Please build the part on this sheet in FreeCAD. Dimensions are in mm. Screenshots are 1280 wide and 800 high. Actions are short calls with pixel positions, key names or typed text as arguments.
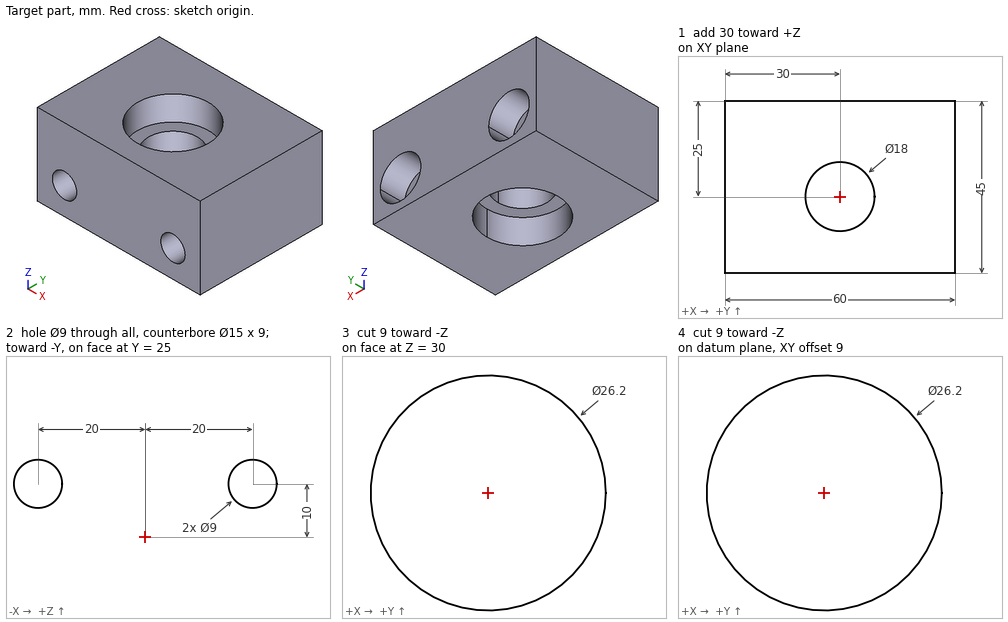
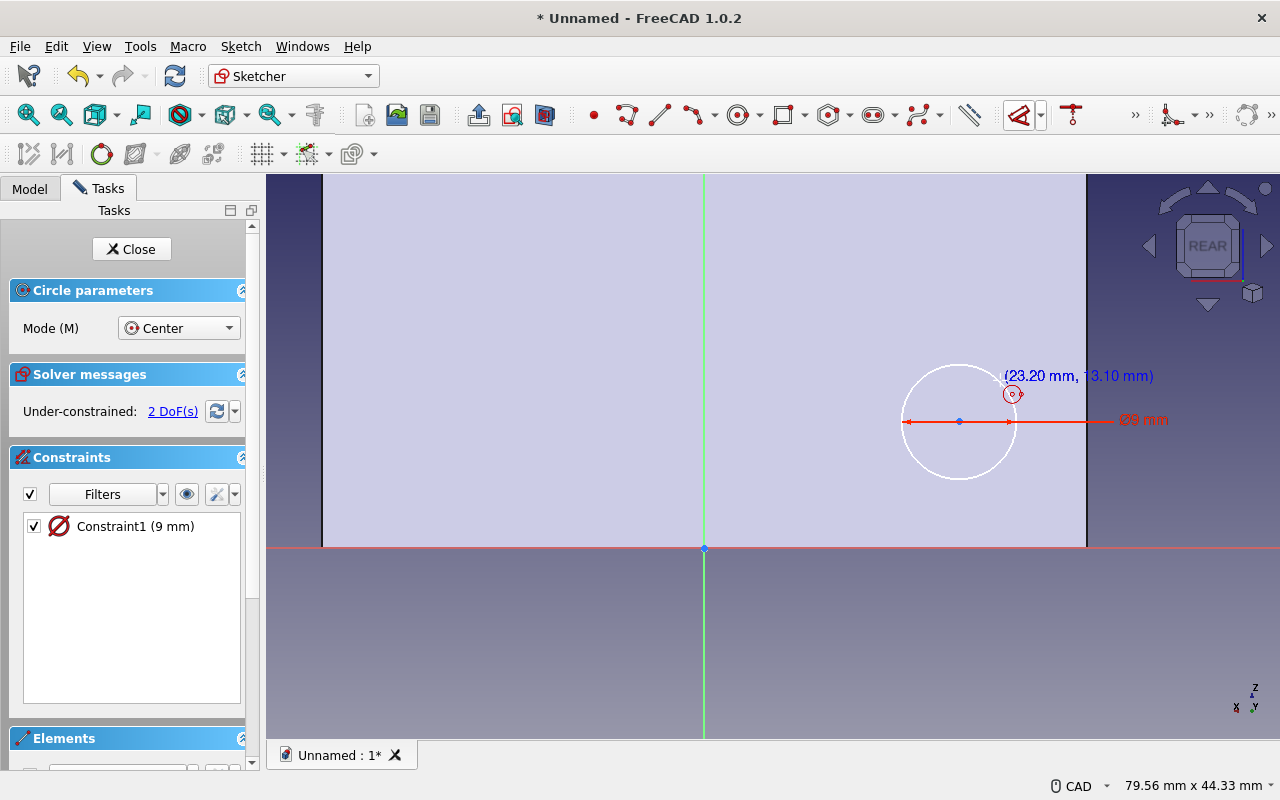
click(449, 421)
move(490, 380)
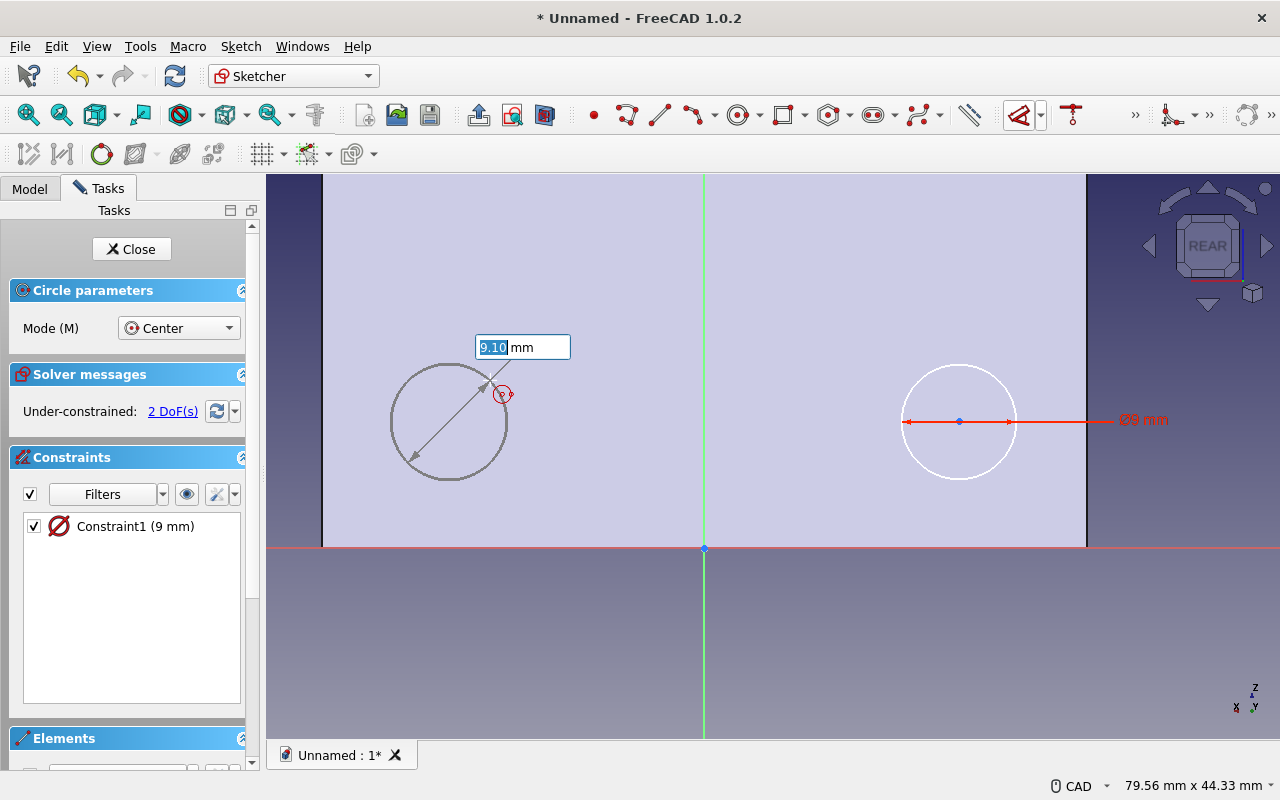
text(9)
key(Return)
key(Escape)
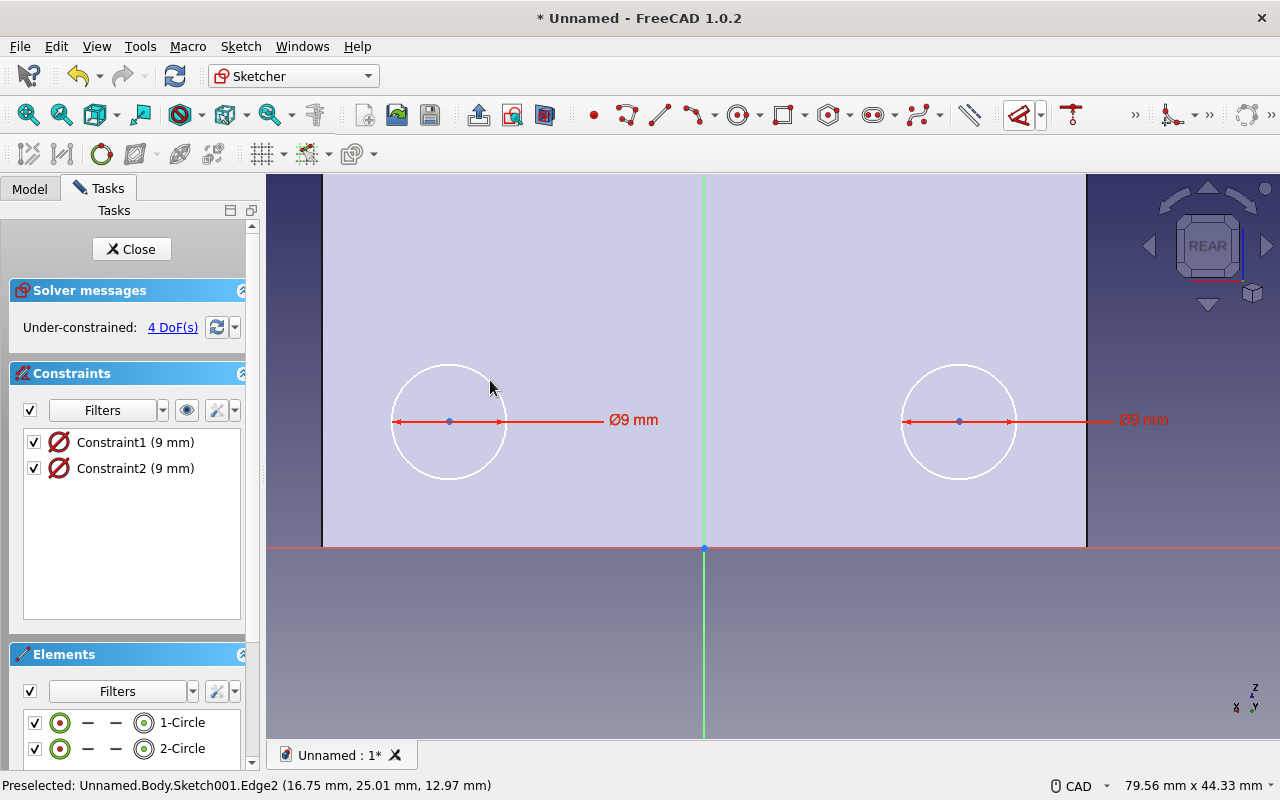
click(959, 422)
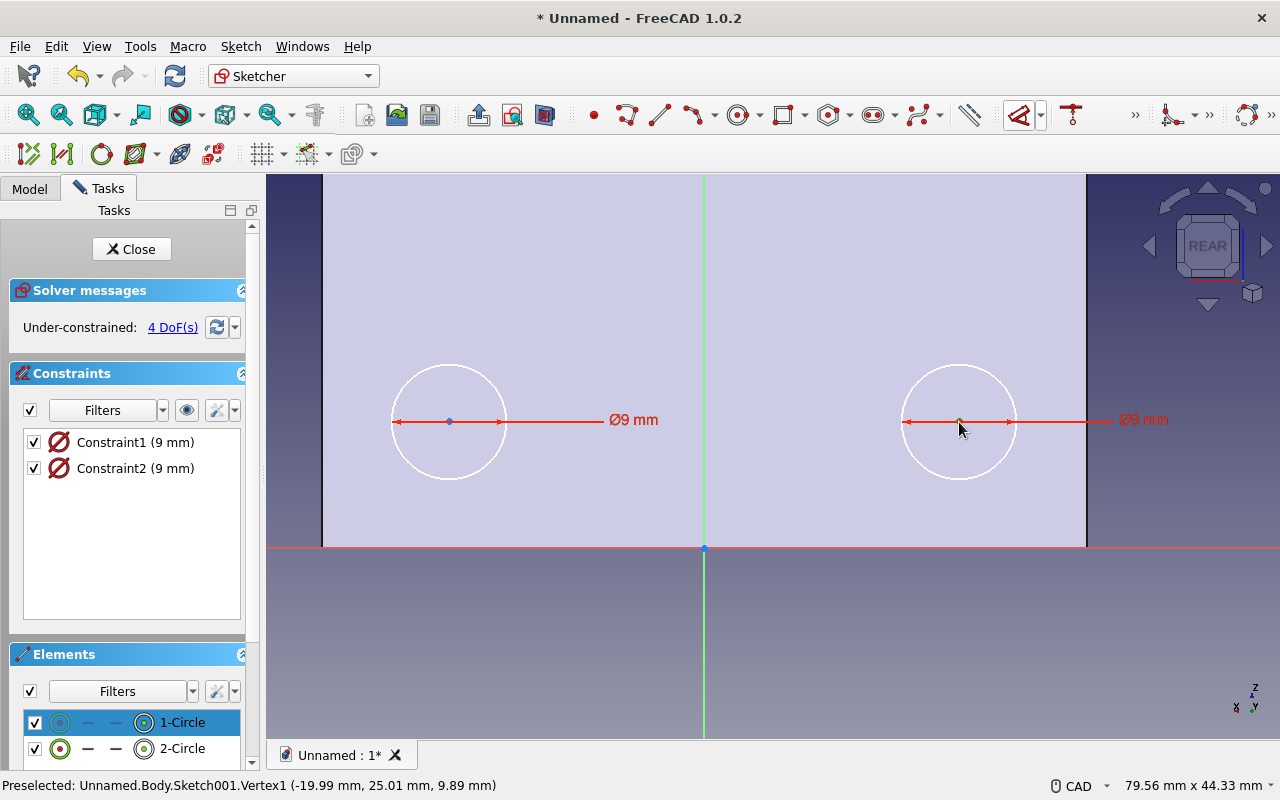
click(449, 422)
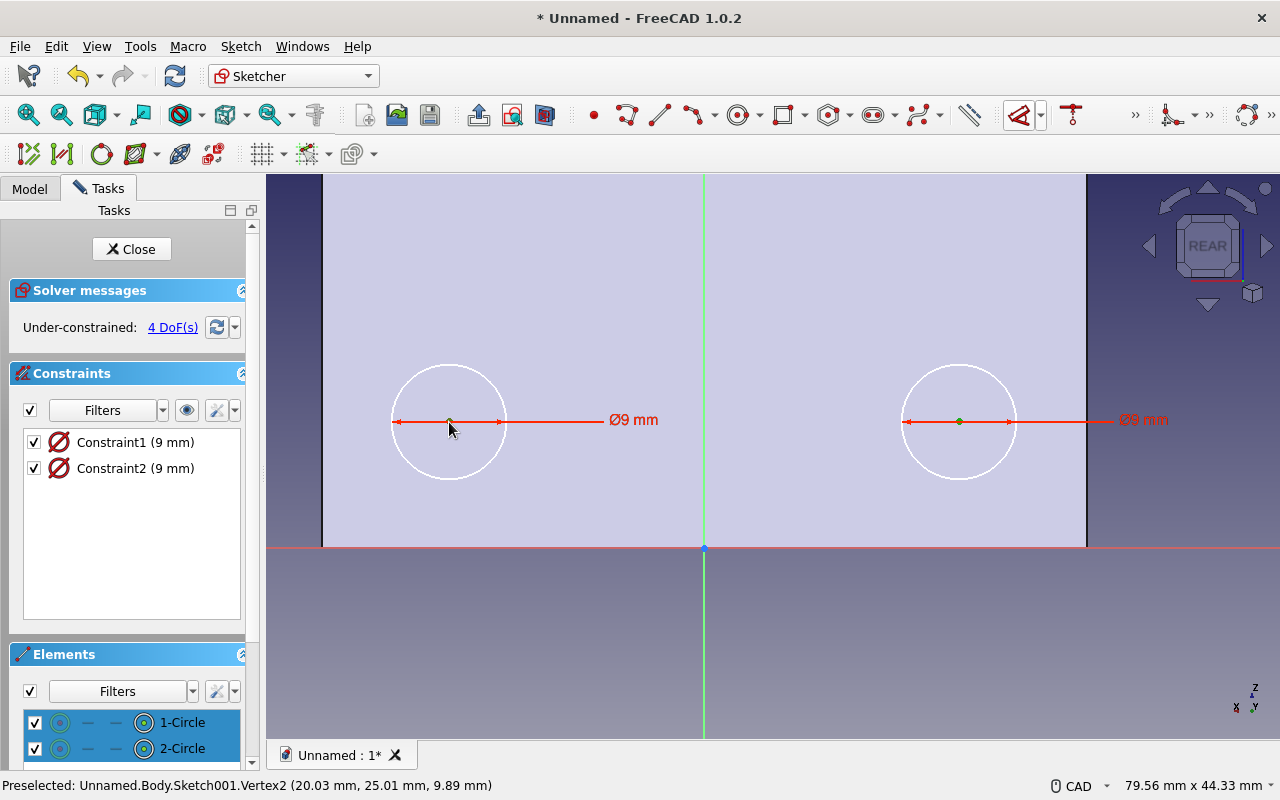
key(h)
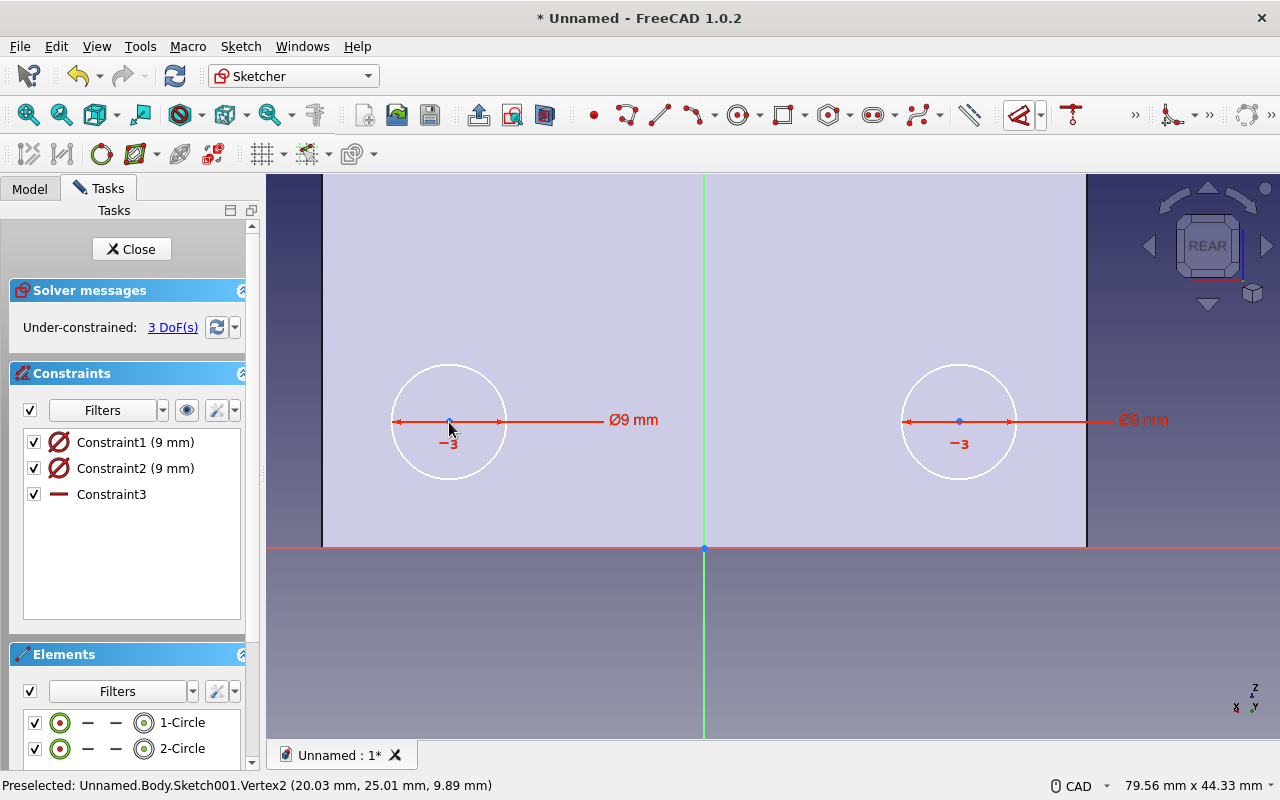
click(959, 422)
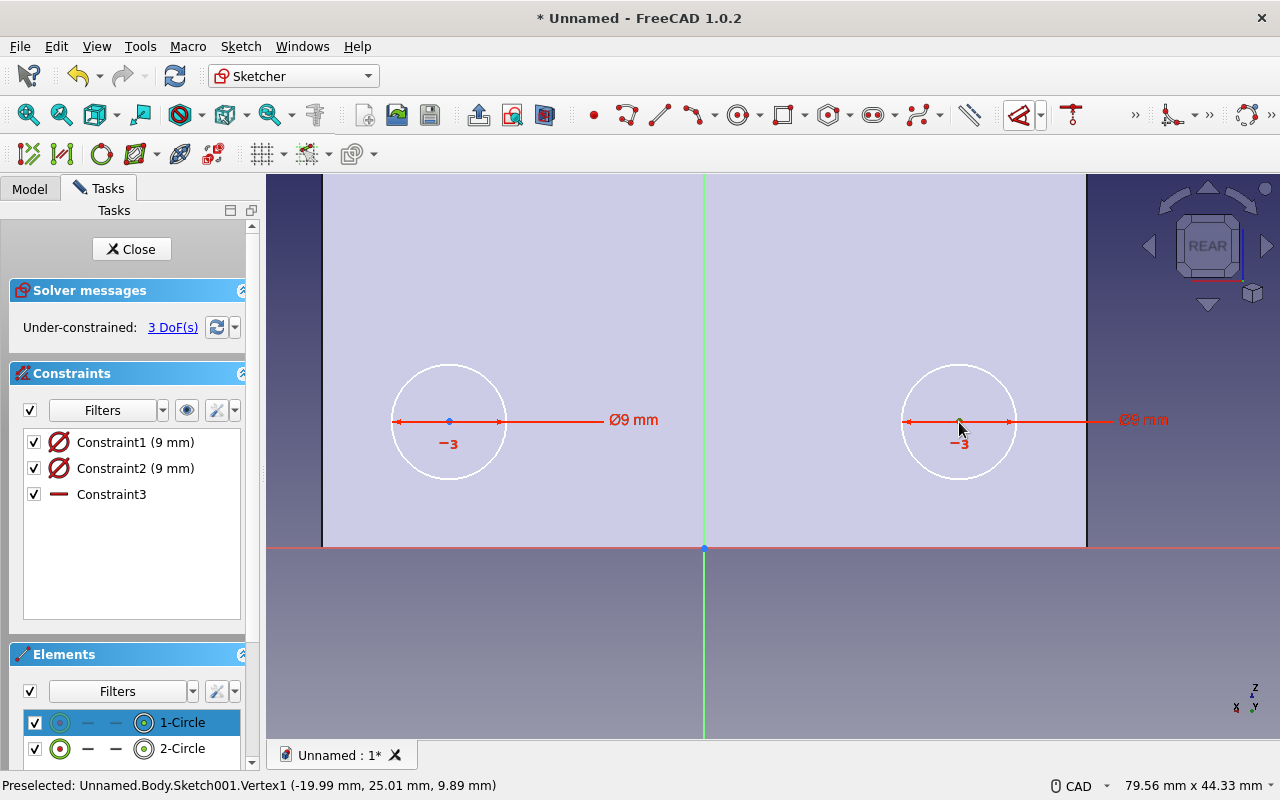
key(l)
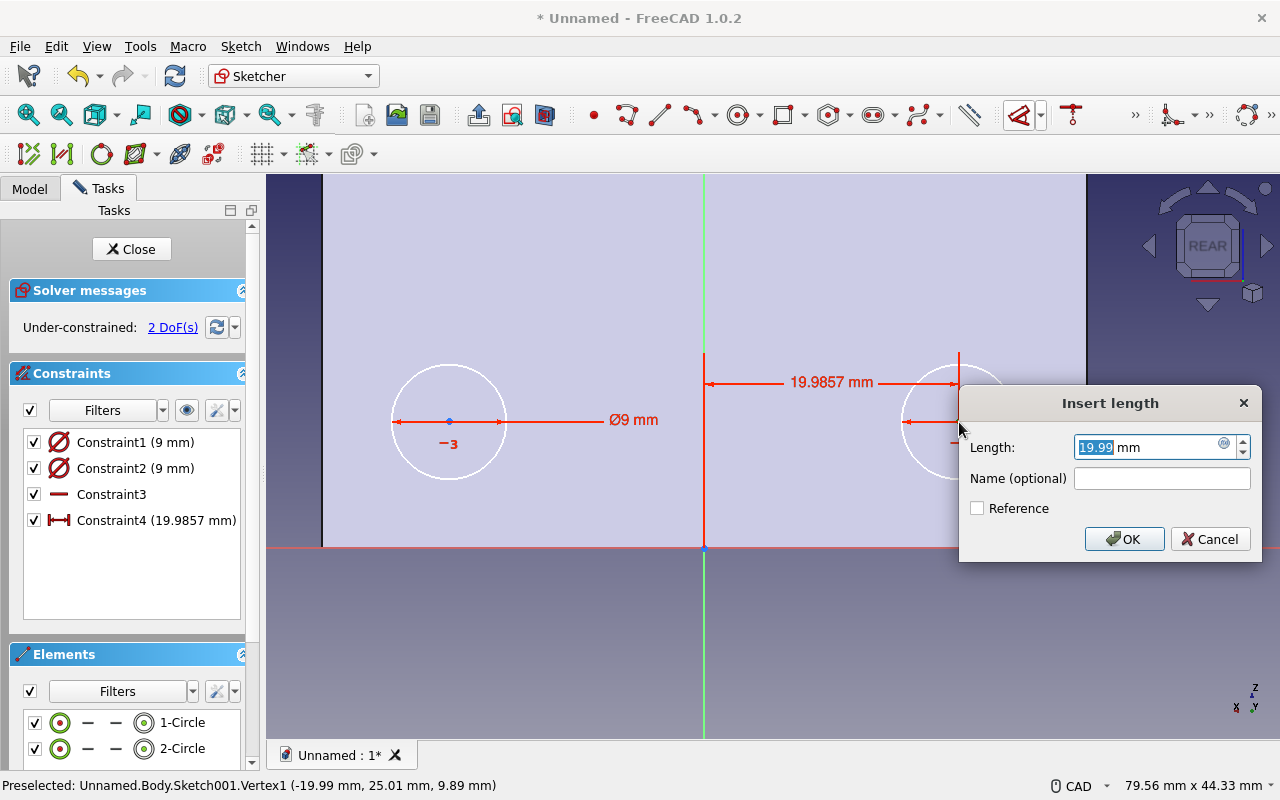
text(20)
key(Return)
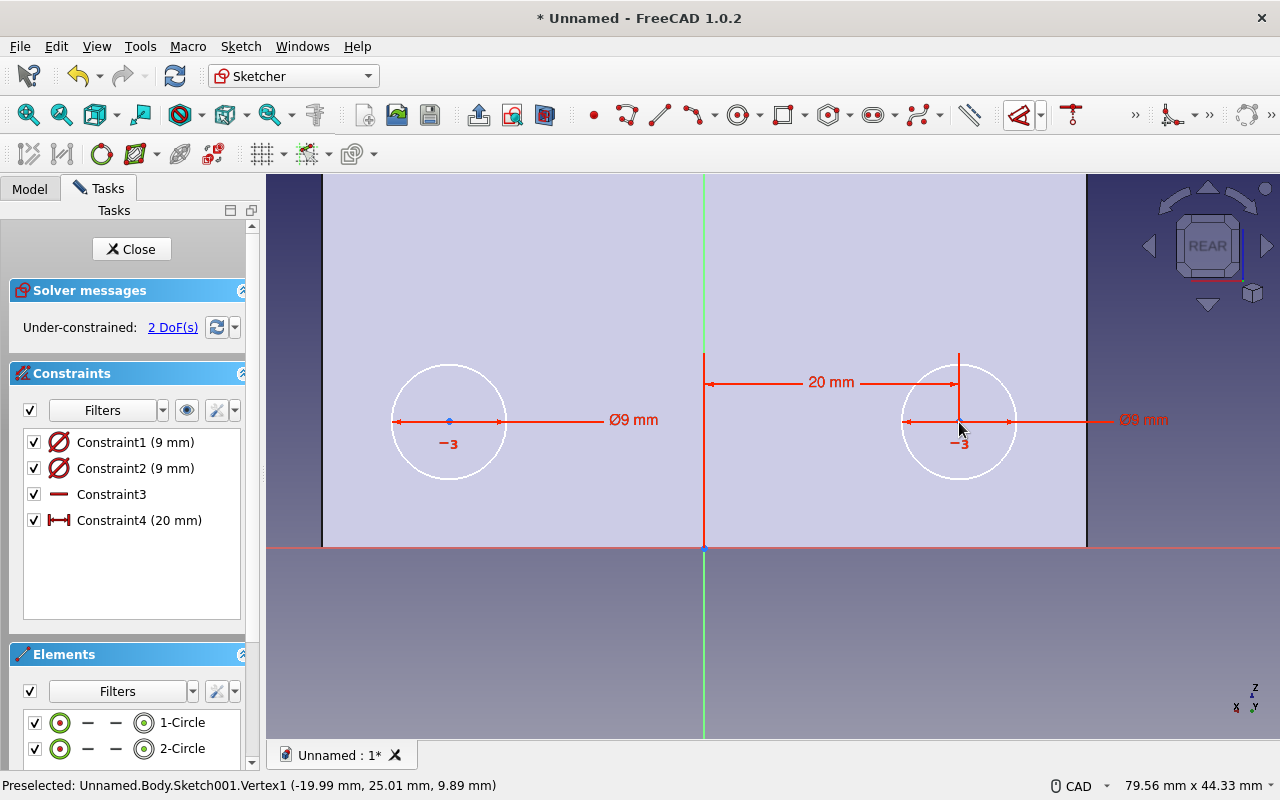
click(959, 422)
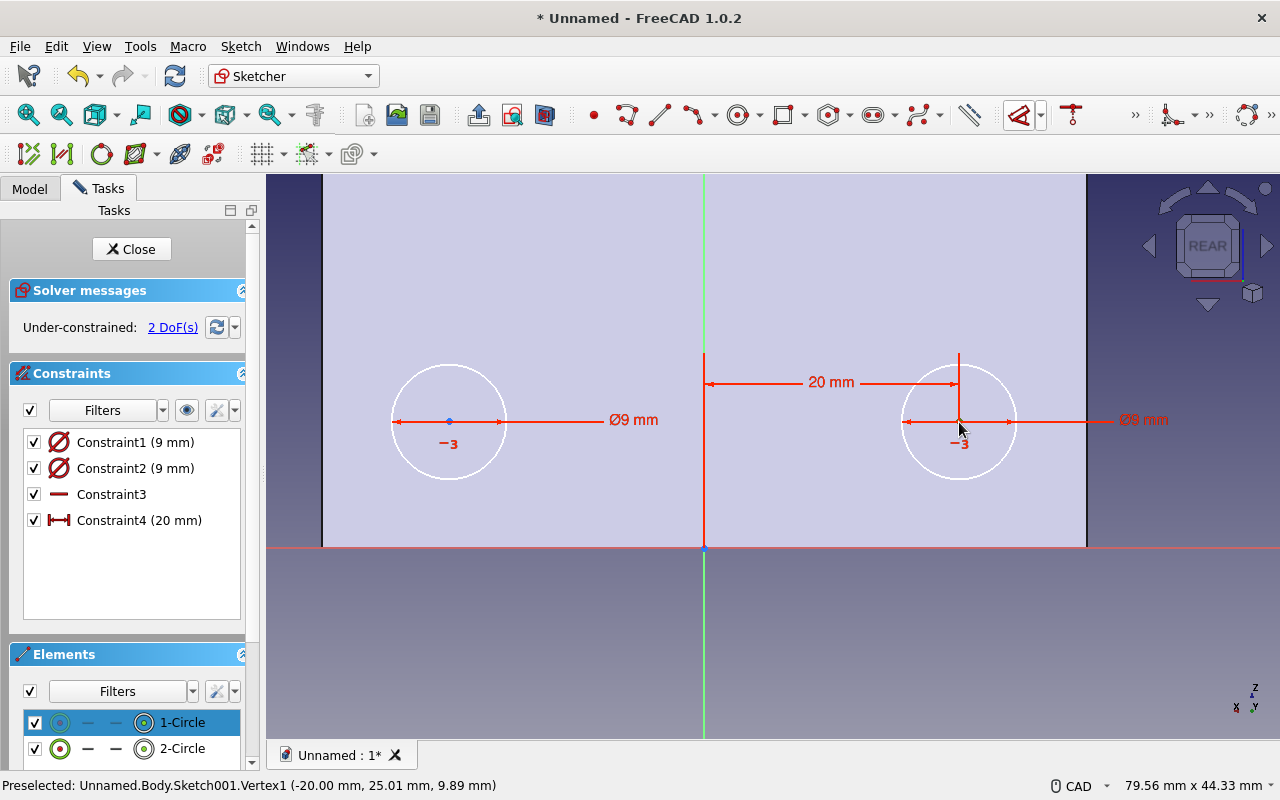
click(1040, 116)